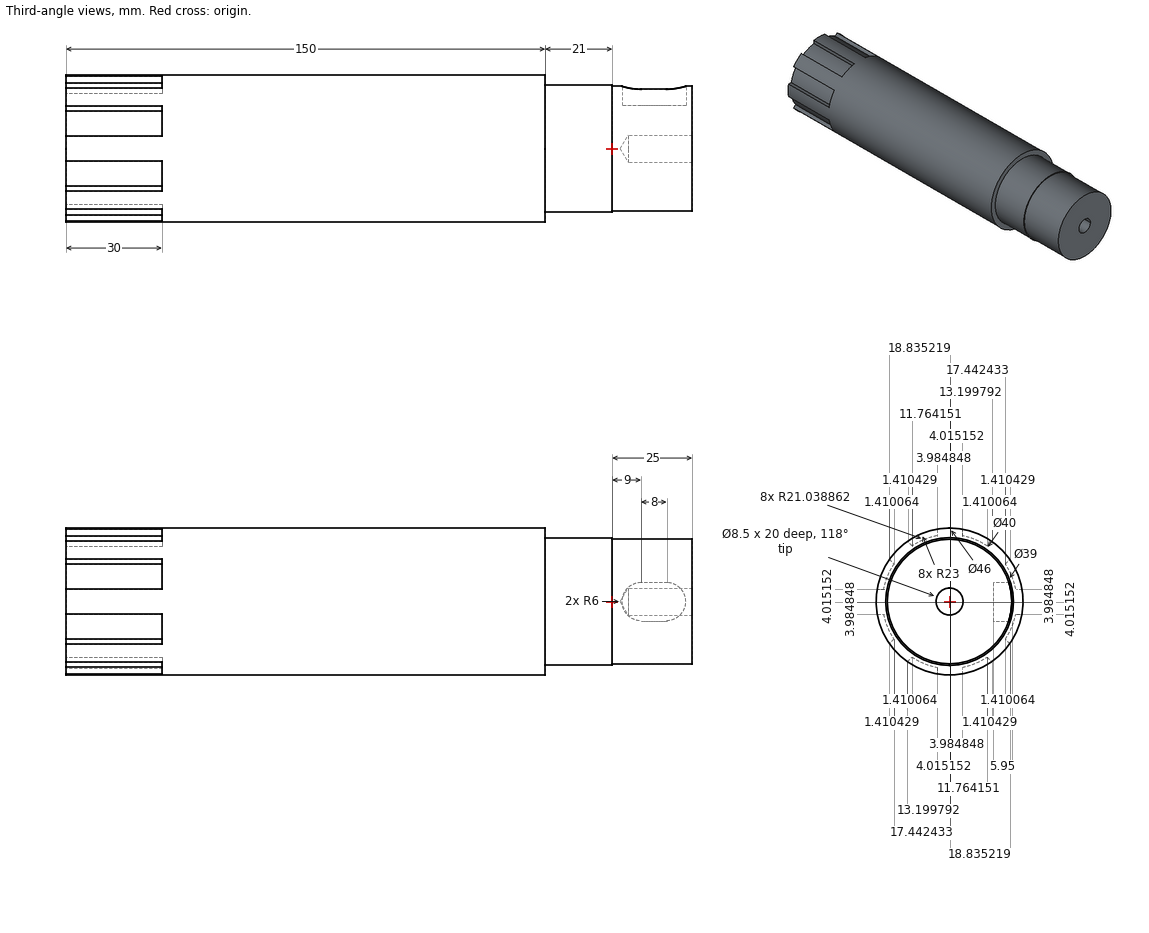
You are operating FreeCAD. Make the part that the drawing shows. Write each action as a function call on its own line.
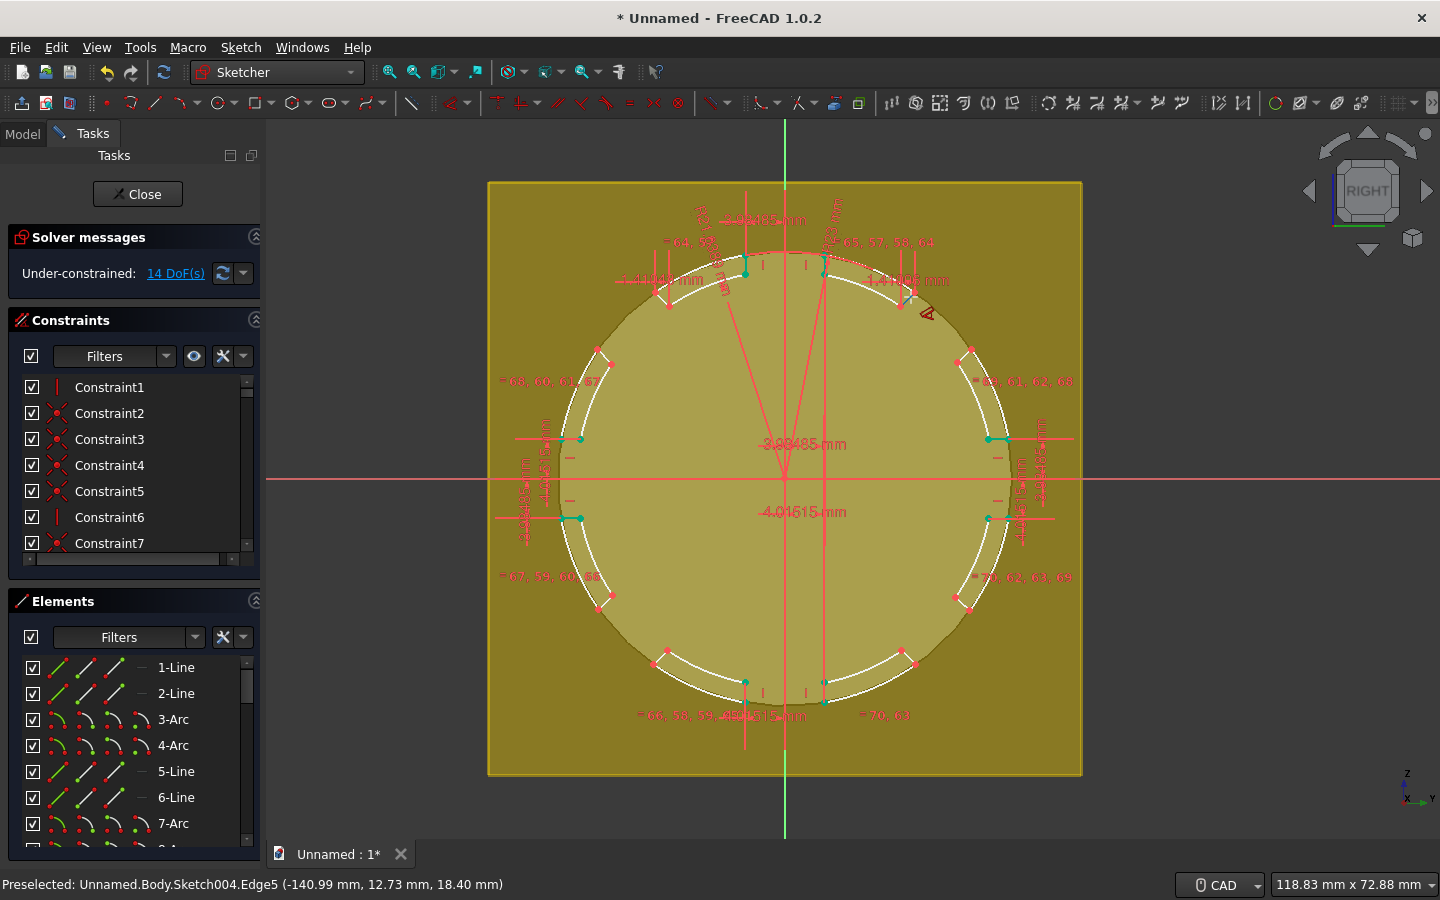
scroll(658, 660, up, 6)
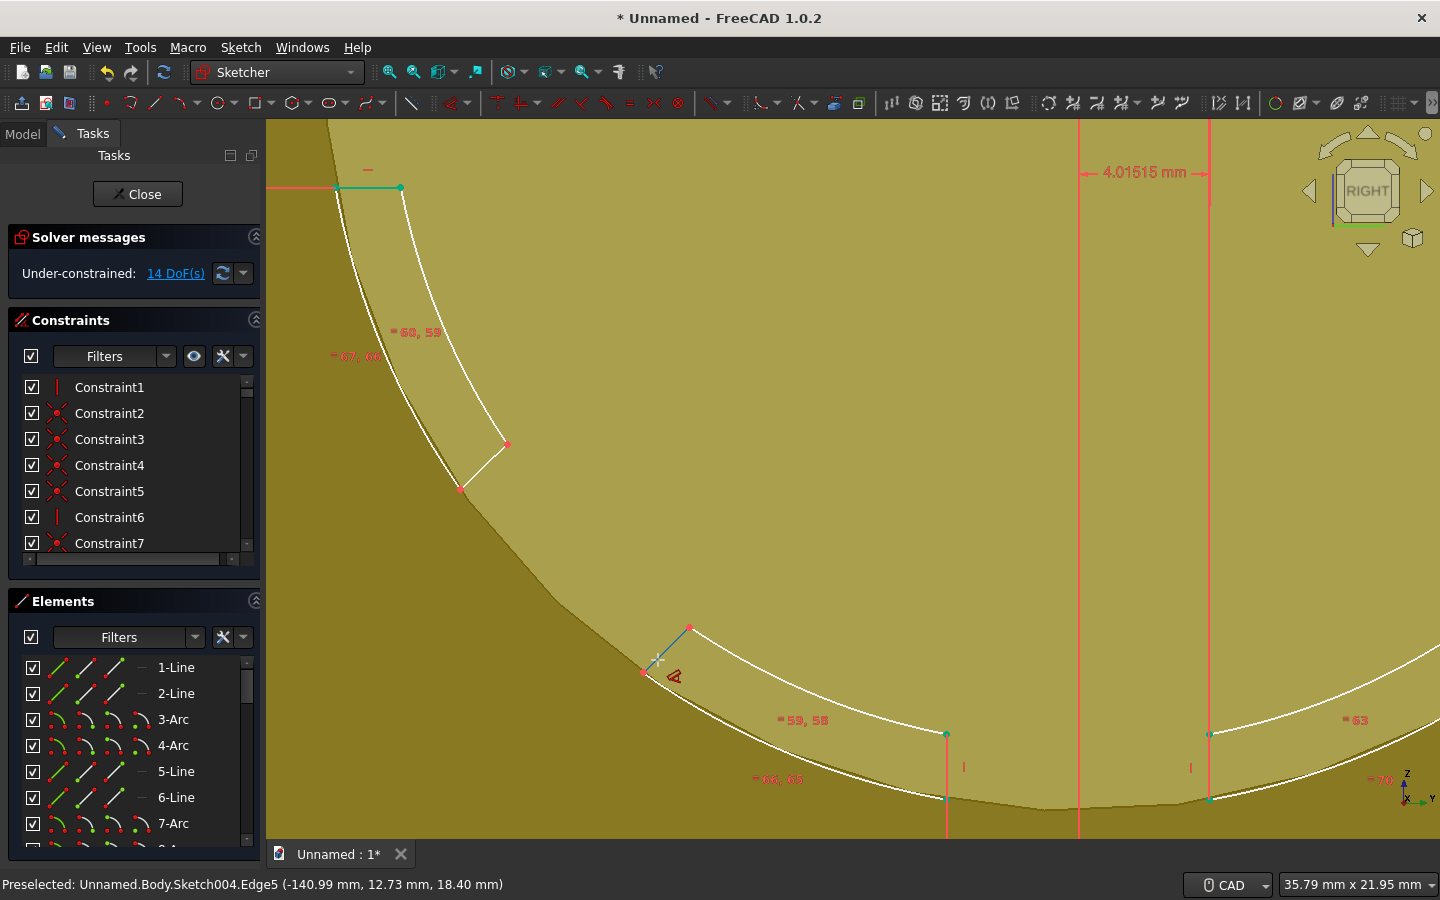
click(657, 659)
click(666, 707)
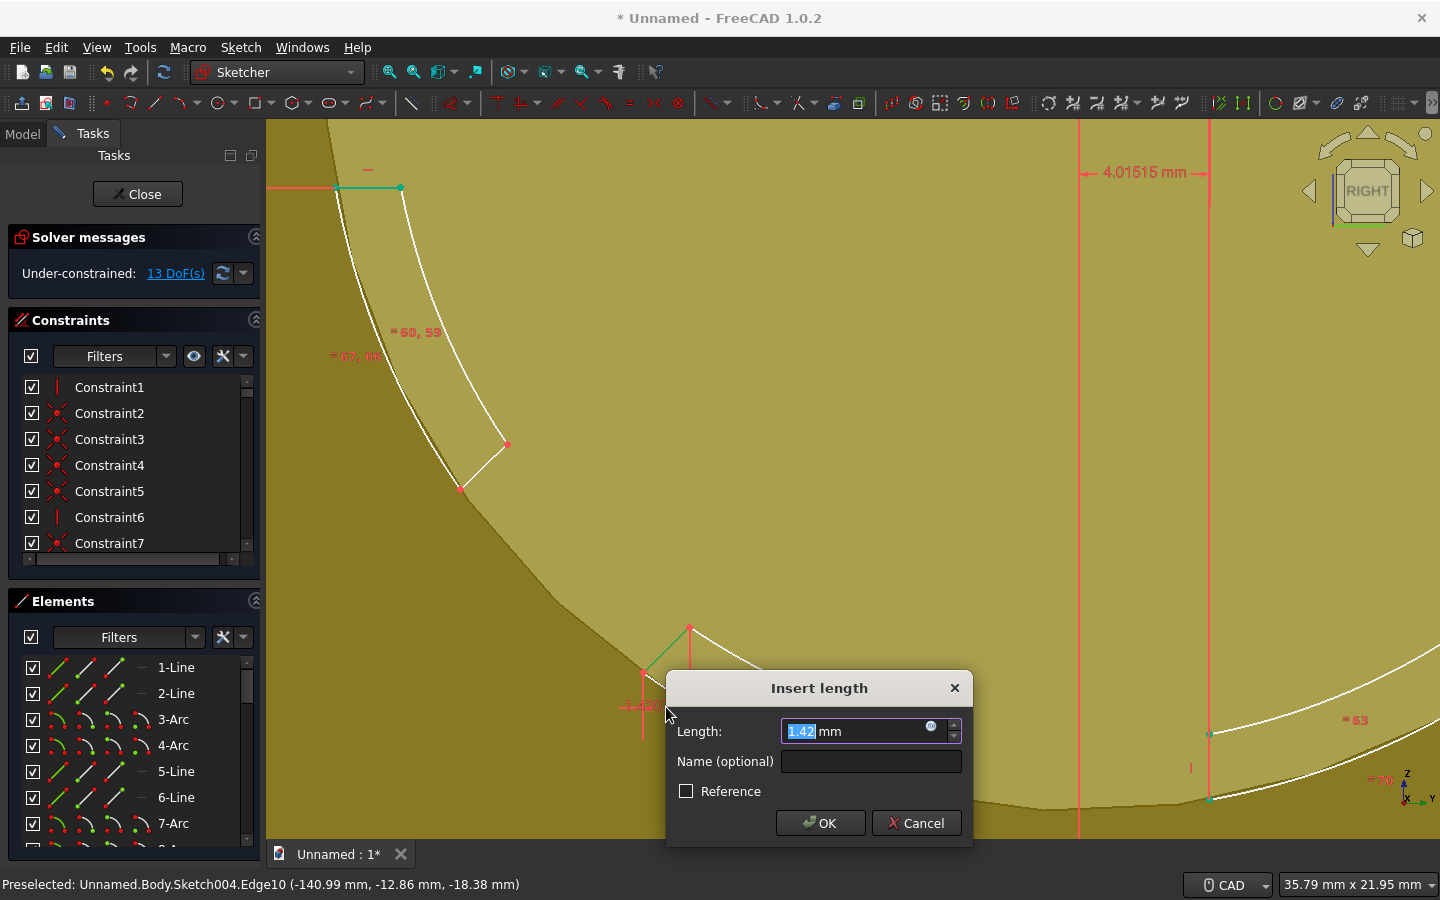
text(1.410064)
key(Return)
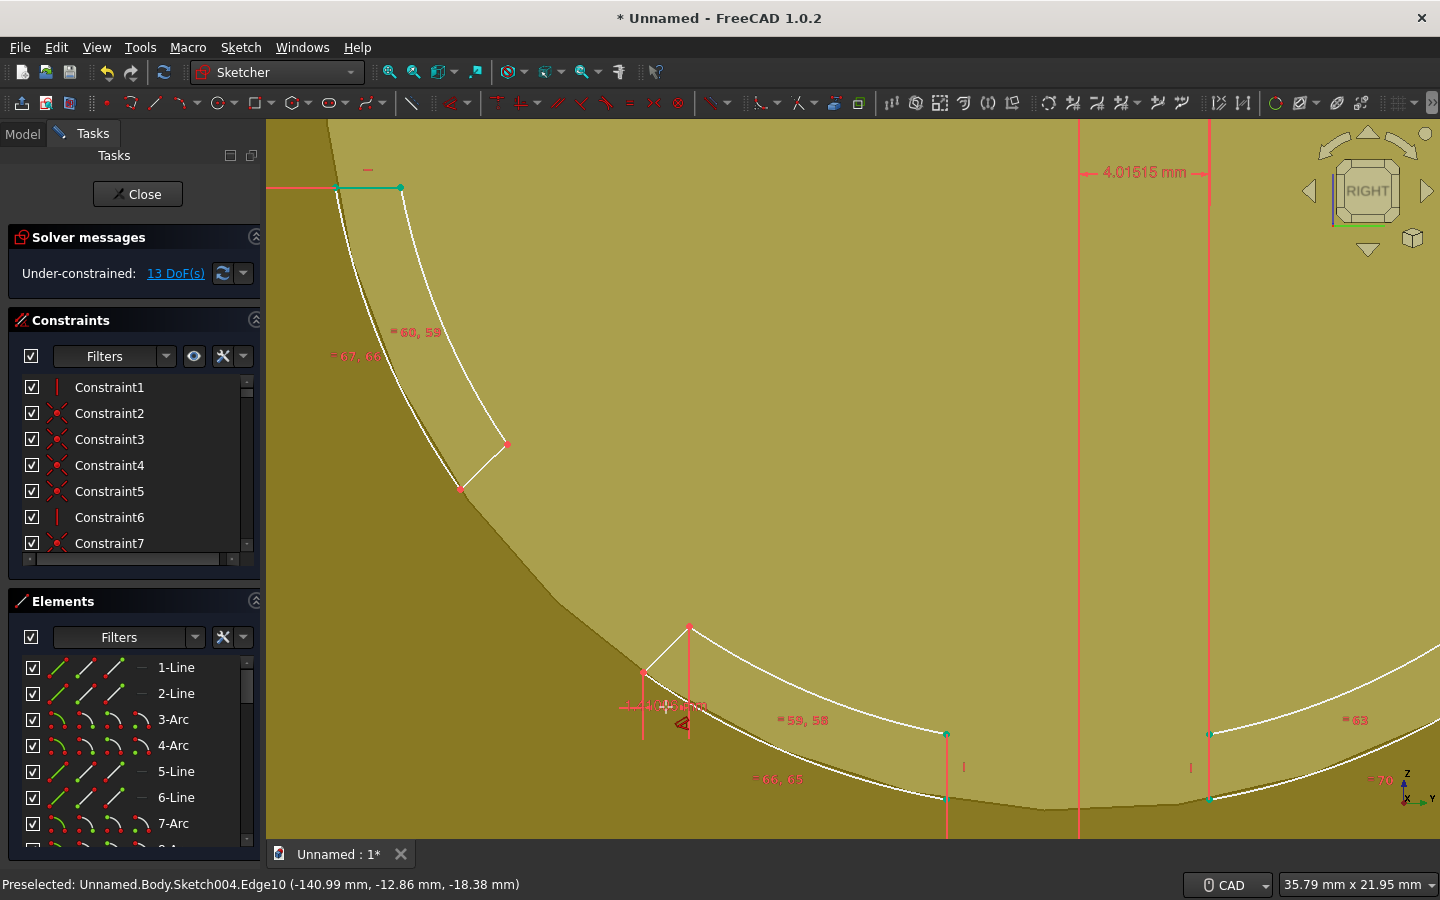
click(493, 458)
click(484, 524)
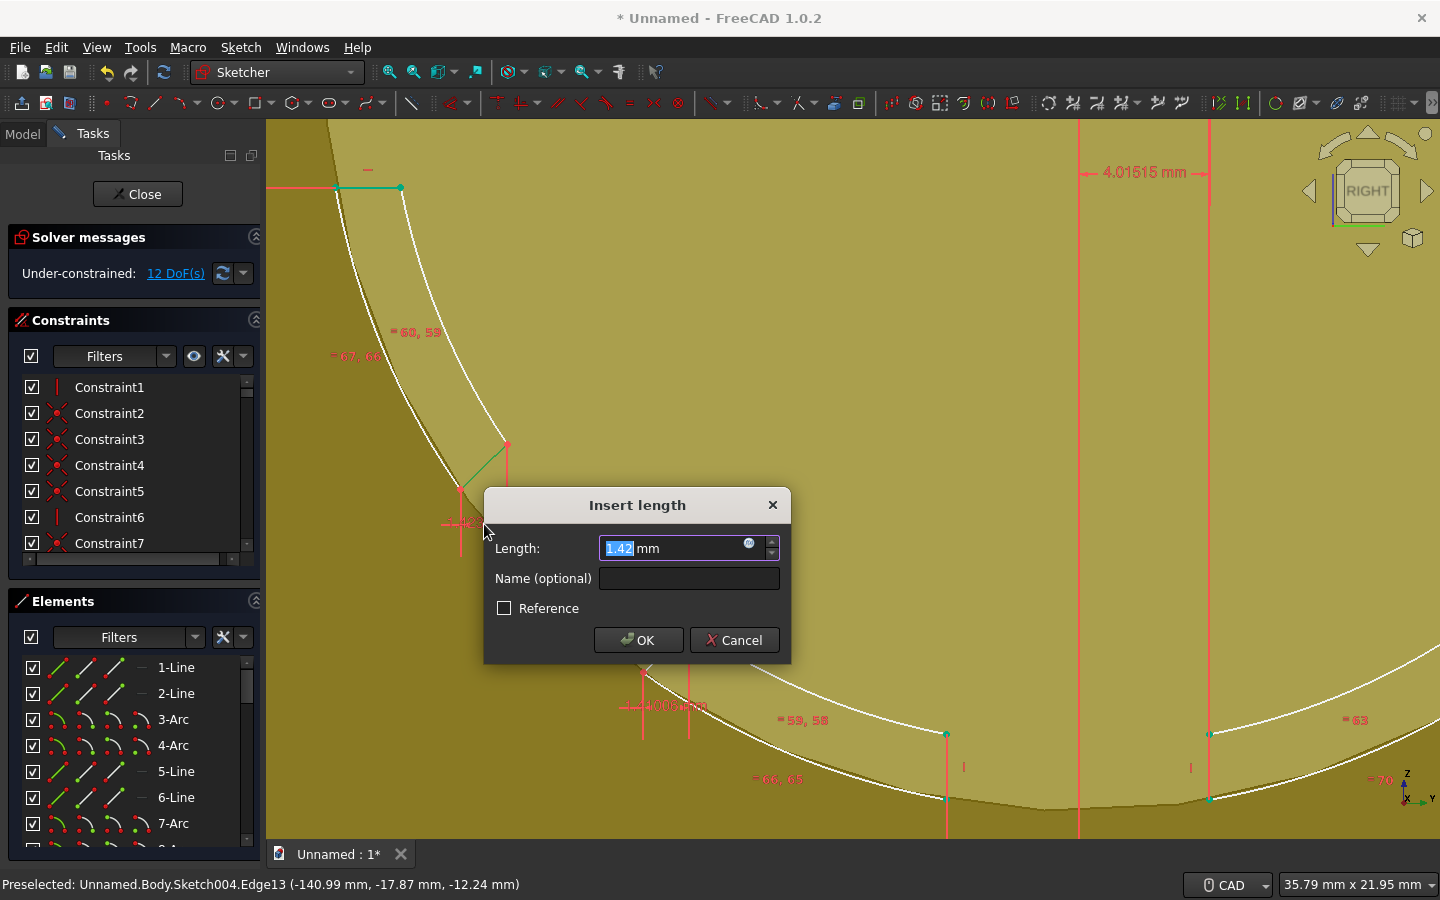
text(1.410429)
key(Return)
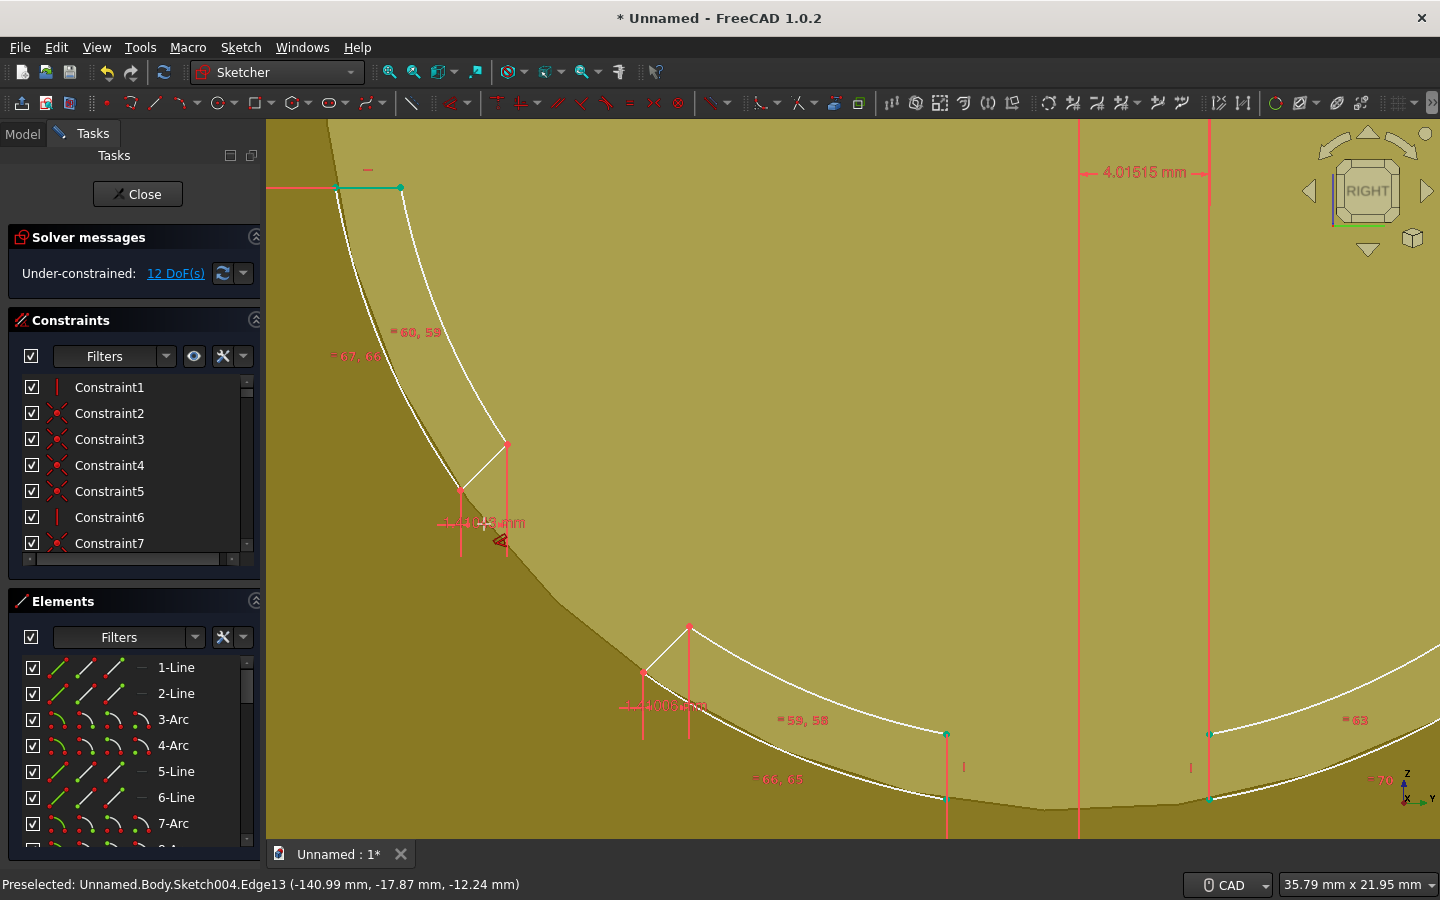
scroll(658, 661, down, 6)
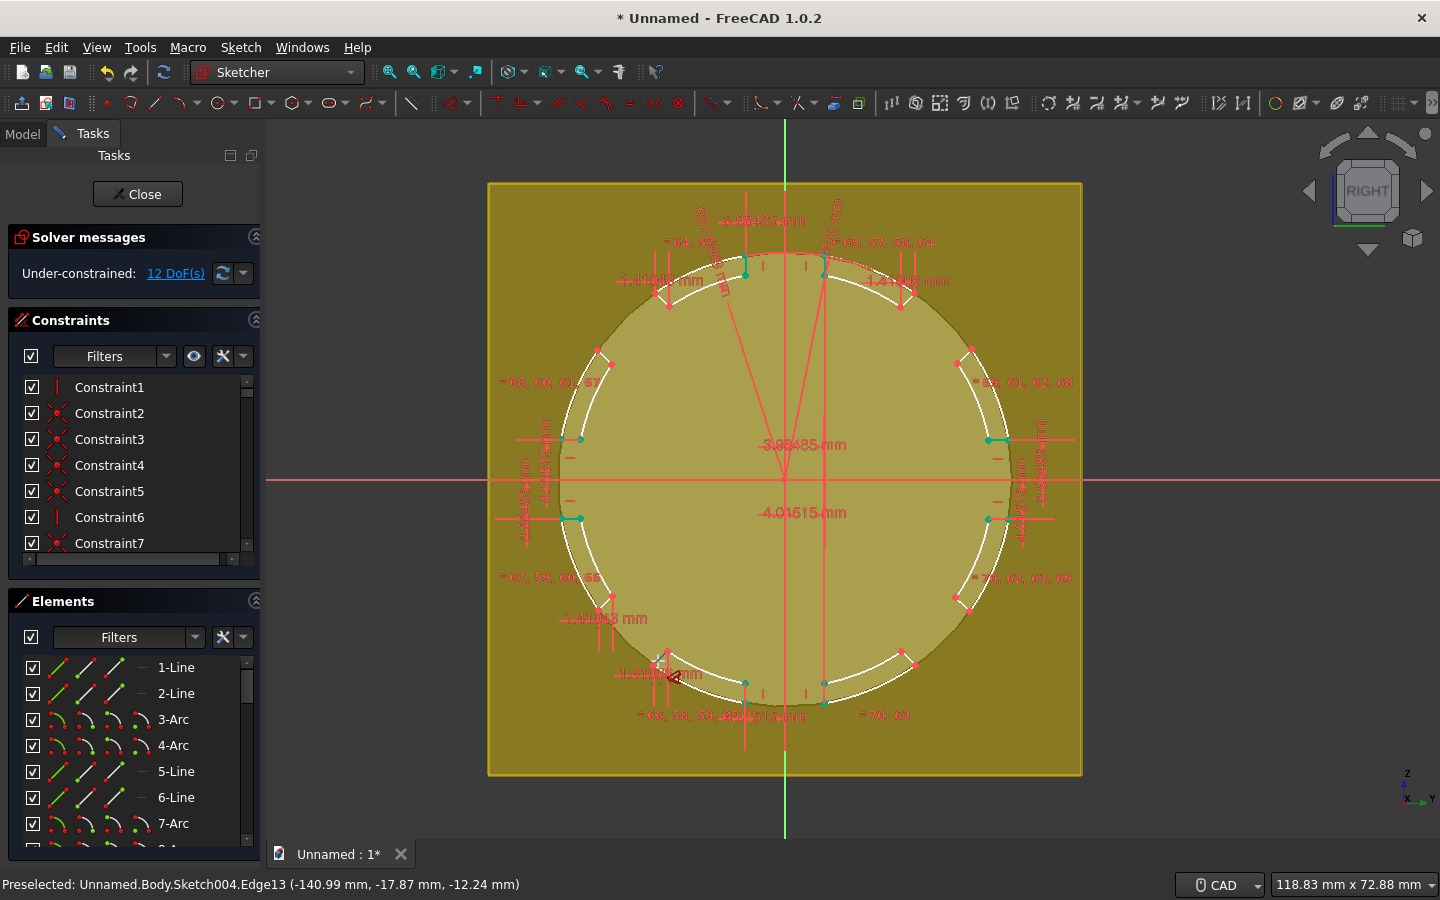
scroll(602, 355, up, 6)